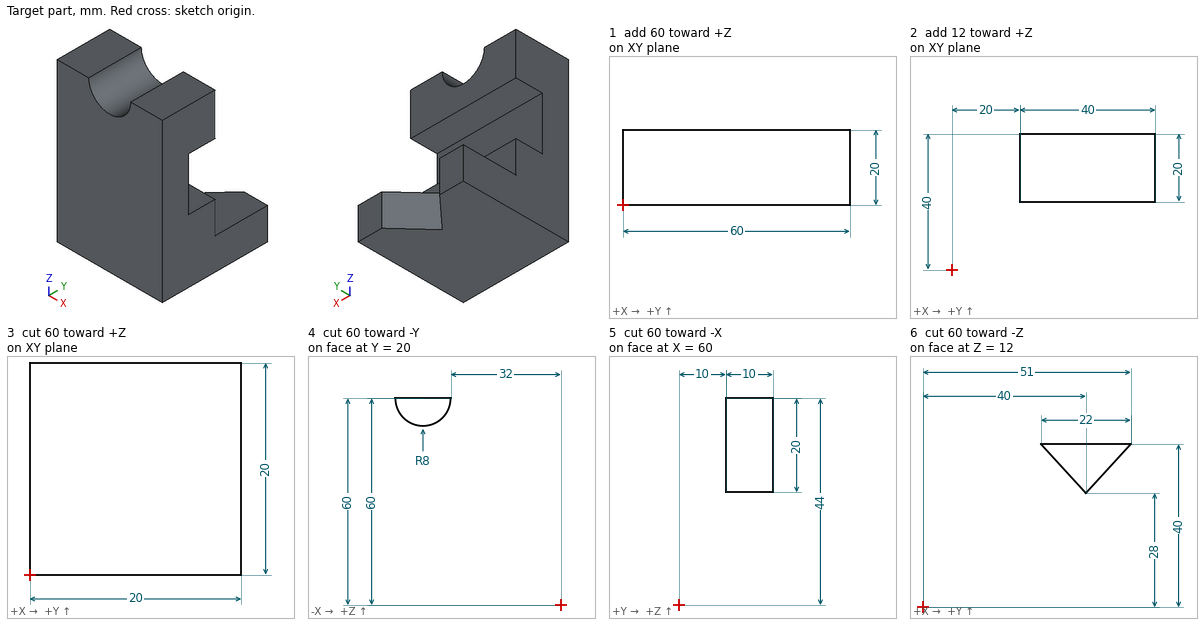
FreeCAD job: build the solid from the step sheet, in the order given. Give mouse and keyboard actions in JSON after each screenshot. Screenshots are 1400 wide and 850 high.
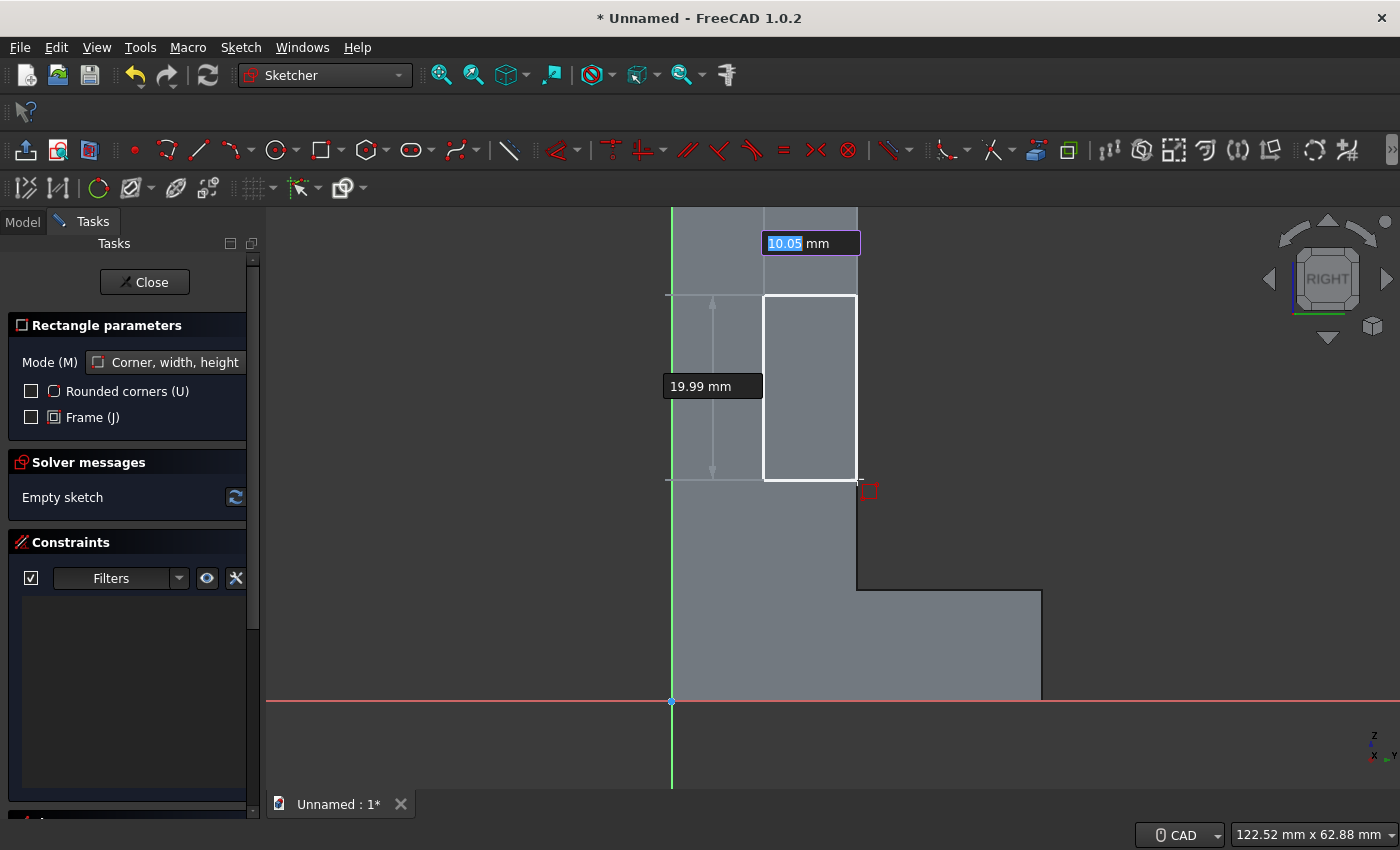
{"action": "type", "text": "10"}
{"action": "key", "text": "Tab"}
{"action": "type", "text": "20"}
{"action": "key", "text": "Return"}
{"action": "key", "text": "Escape"}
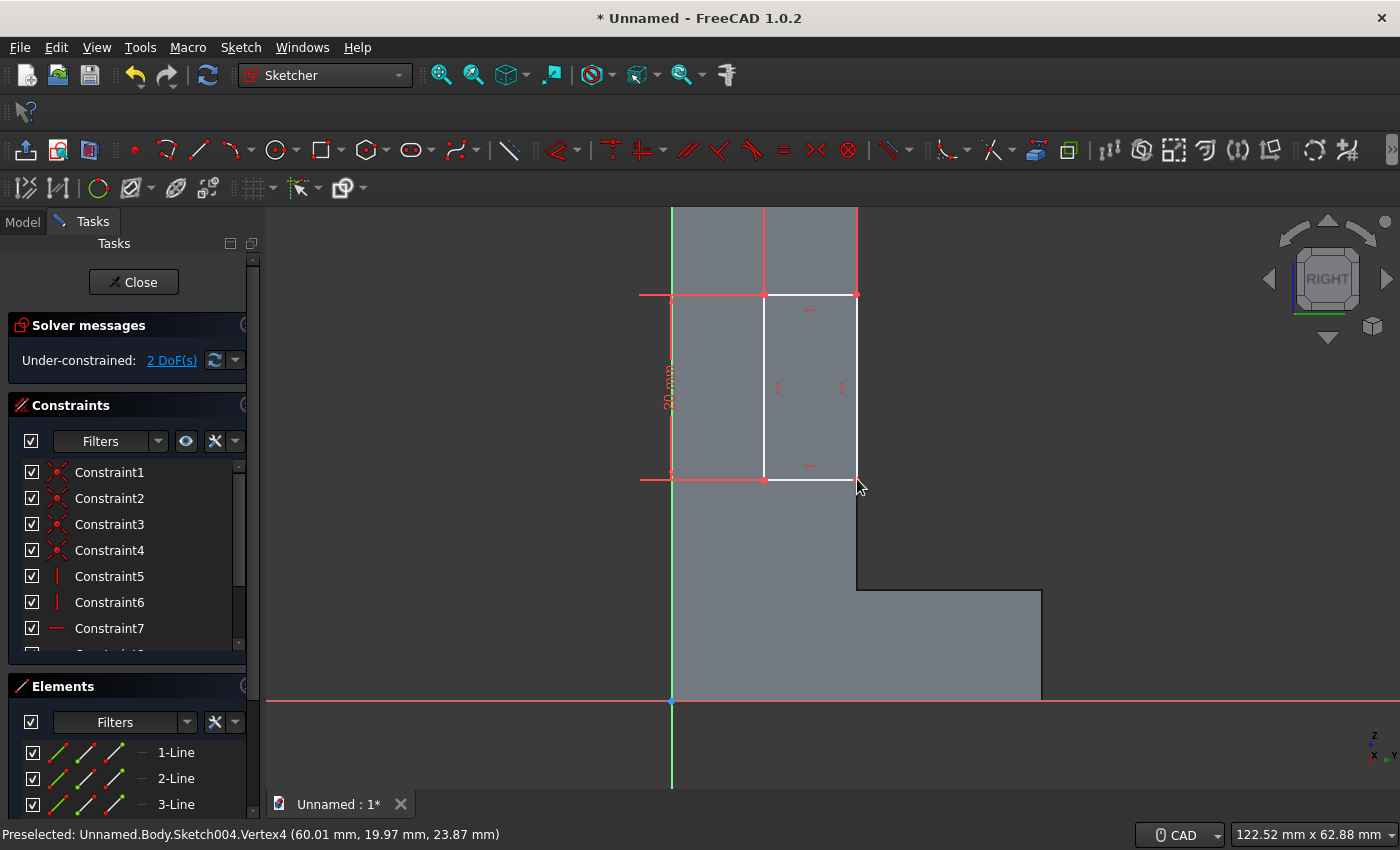
{"action": "left_click", "coordinate": [556, 150]}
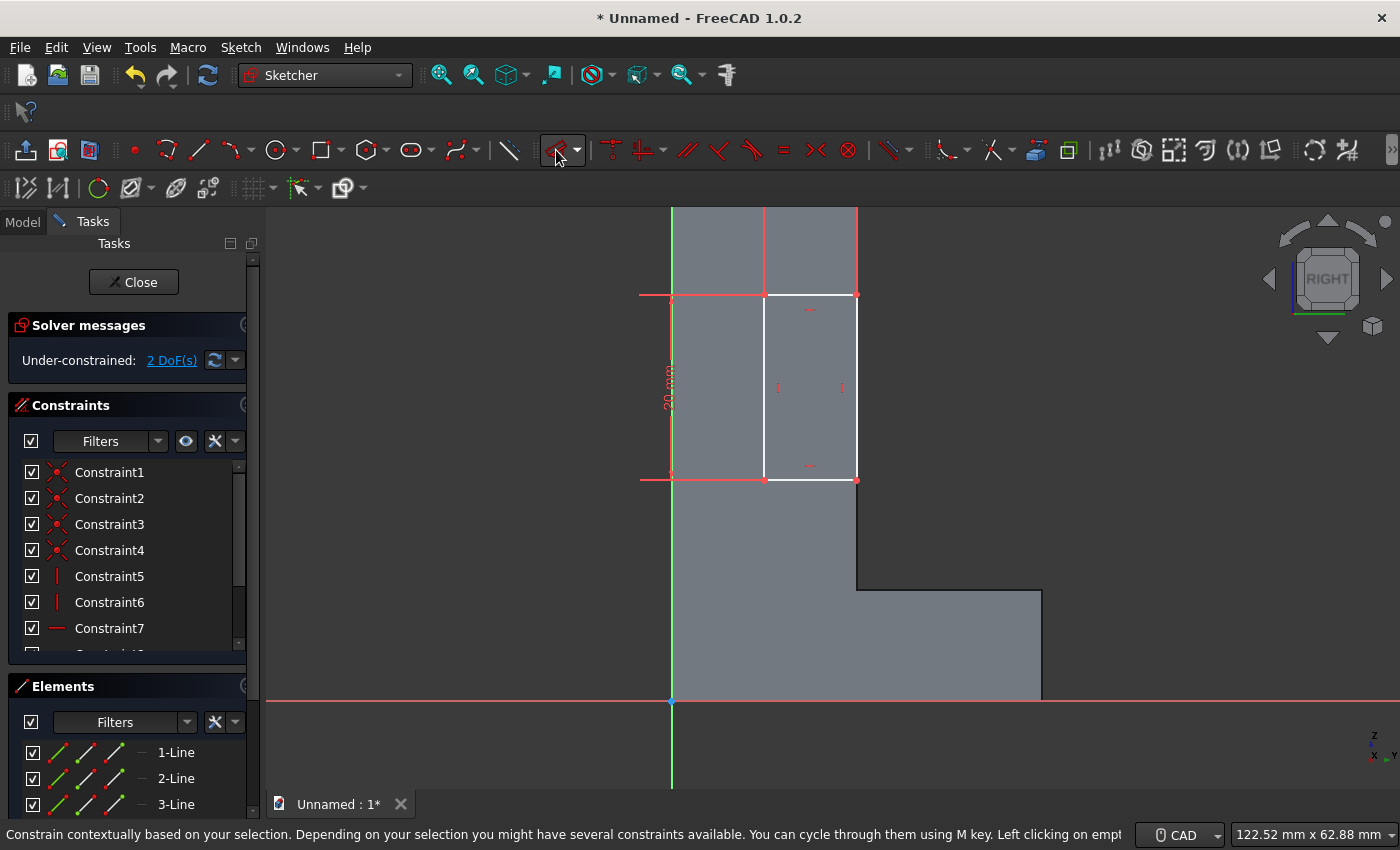
{"action": "left_click", "coordinate": [764, 295]}
{"action": "left_click", "coordinate": [718, 735]}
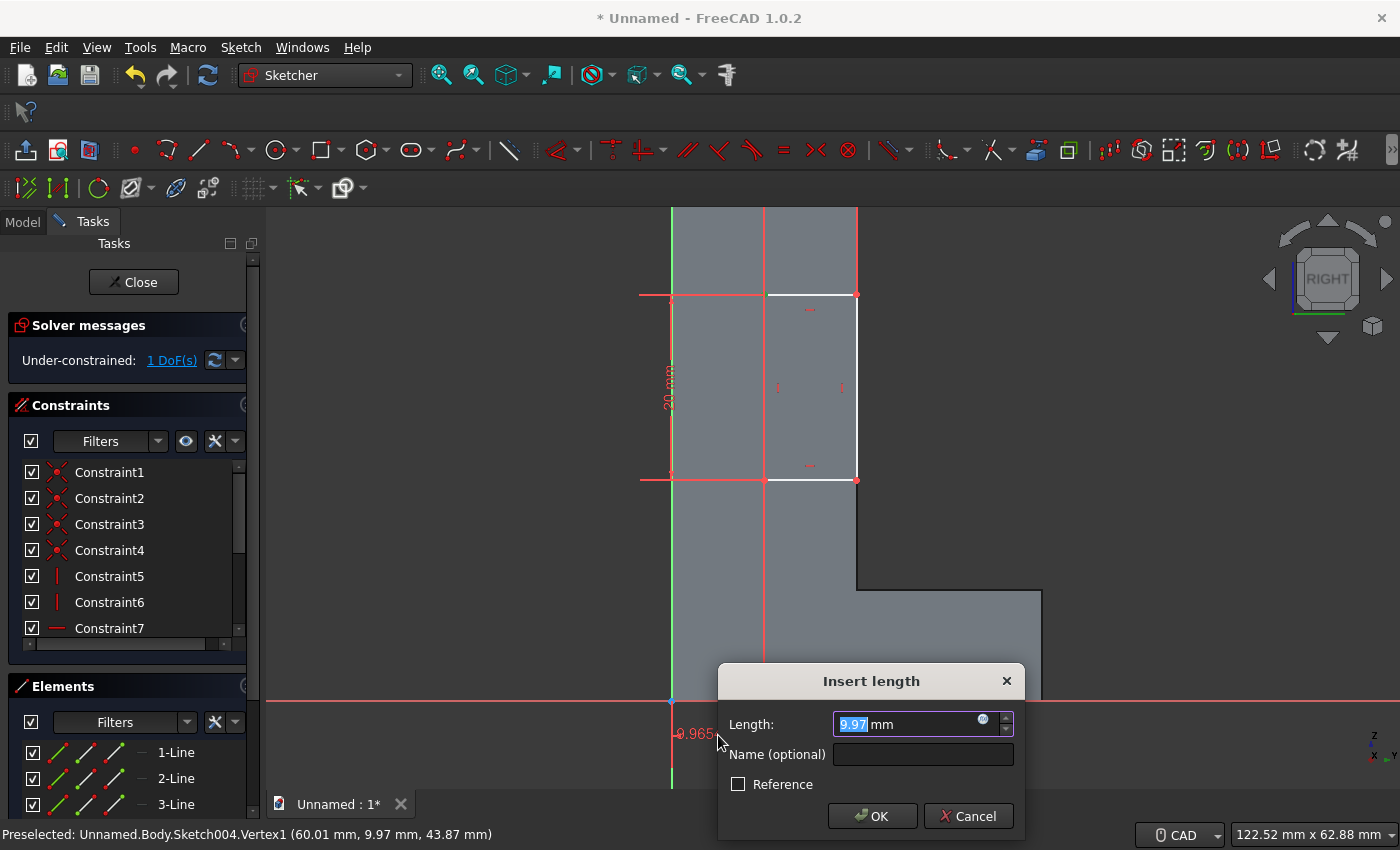
{"action": "type", "text": "10"}
{"action": "key", "text": "Return"}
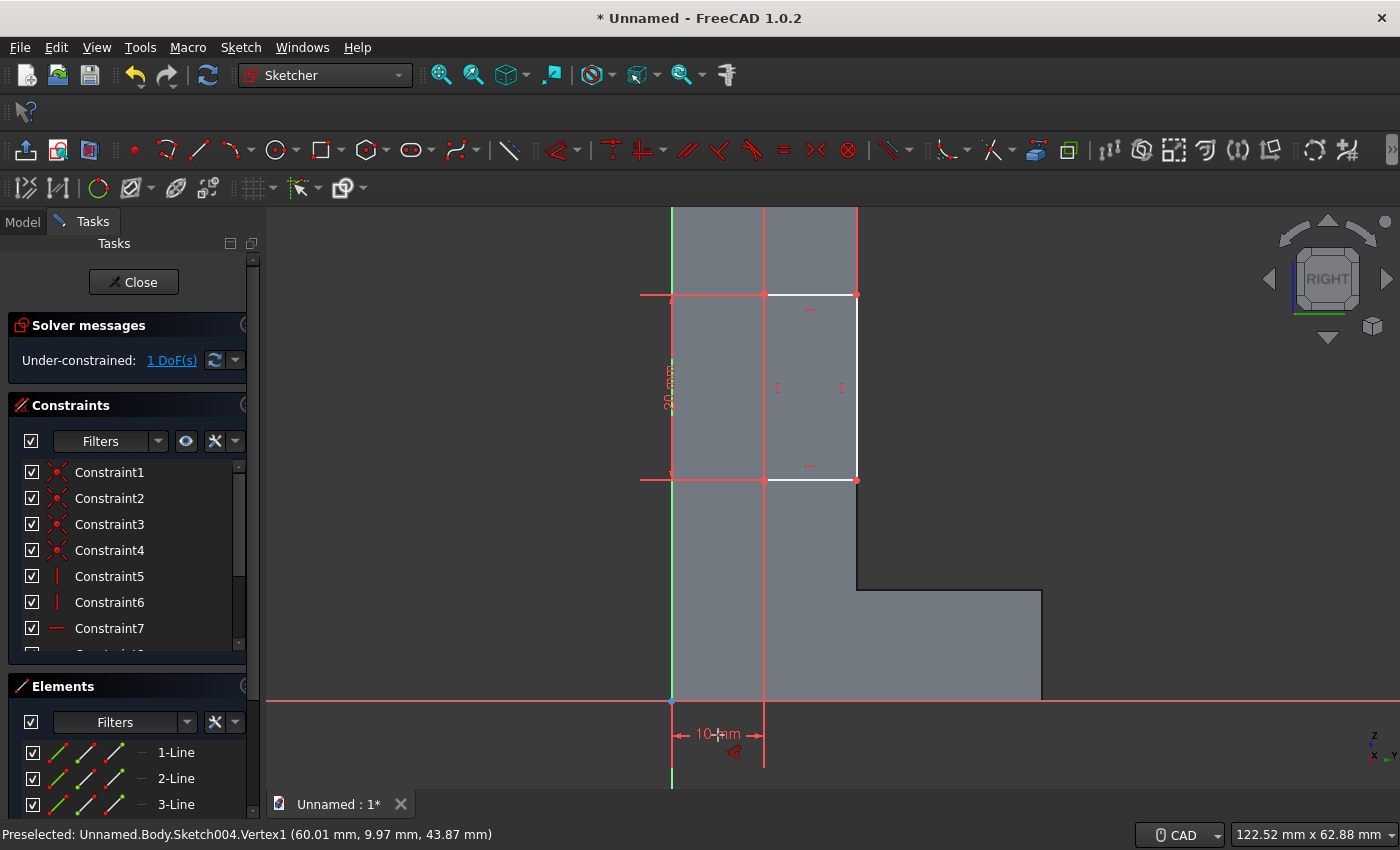
{"action": "left_click", "coordinate": [764, 295]}
{"action": "left_click", "coordinate": [638, 498]}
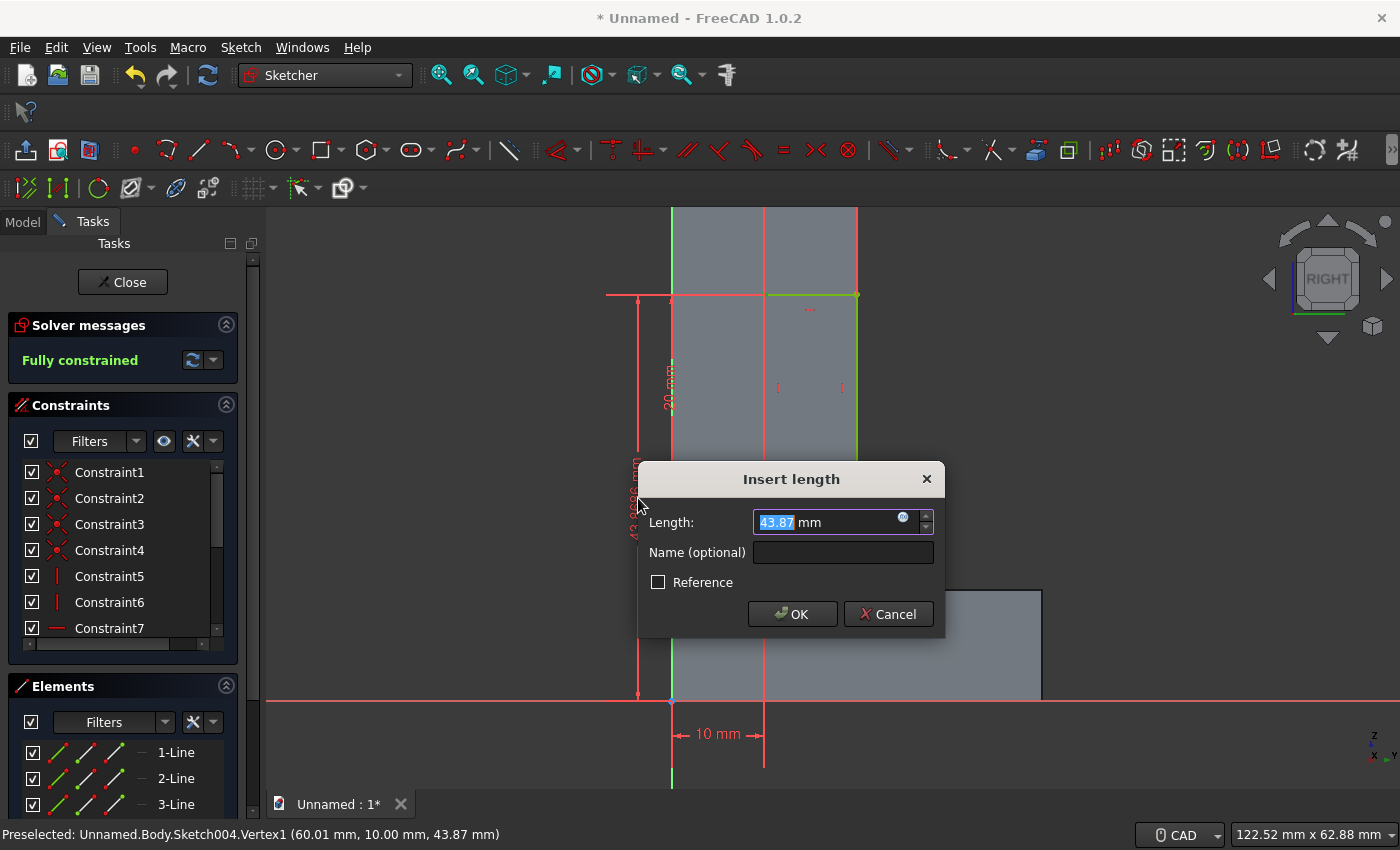
{"action": "type", "text": "44"}
{"action": "key", "text": "Return"}
{"action": "key", "text": "Escape"}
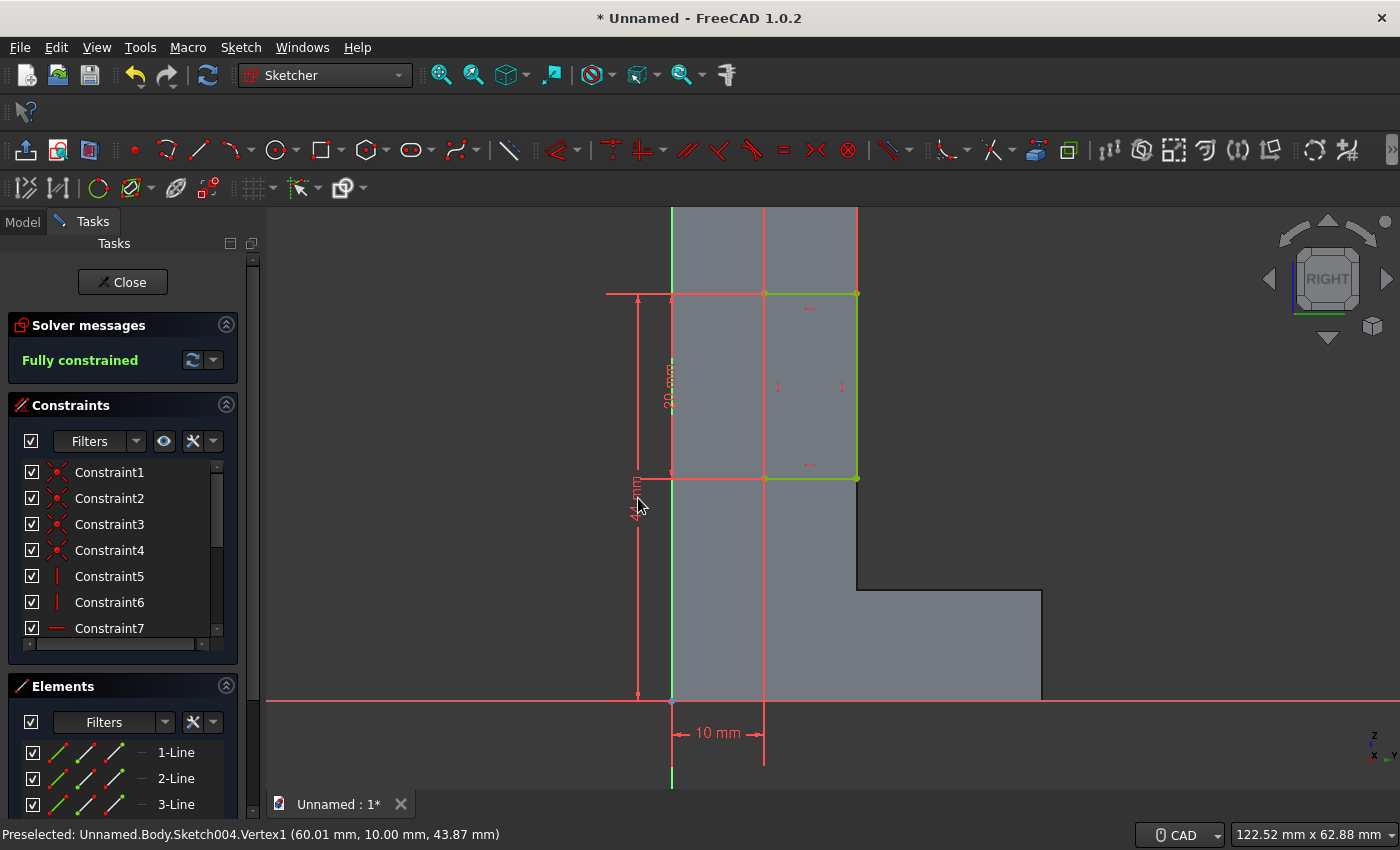
{"action": "left_click", "coordinate": [123, 282]}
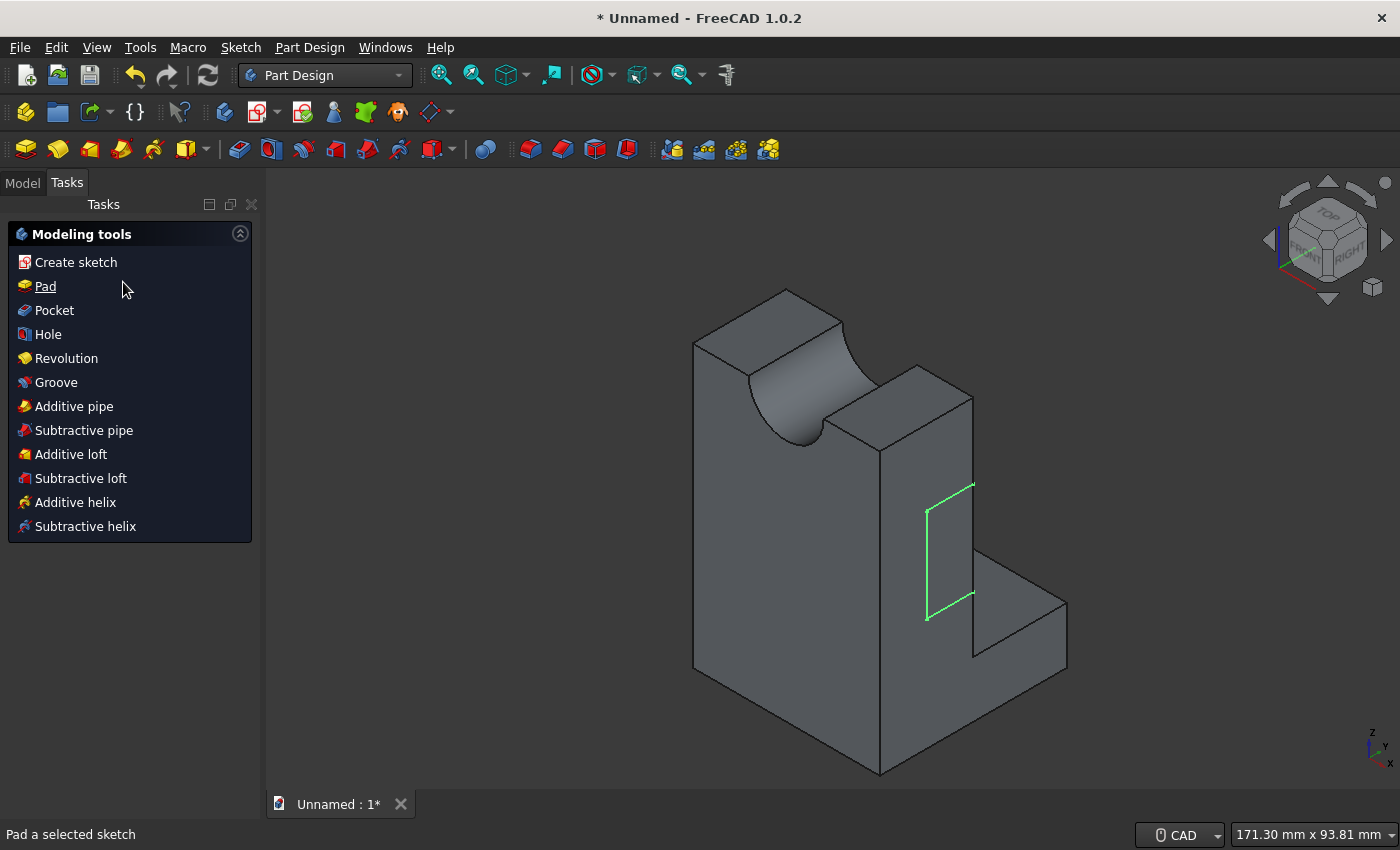
{"action": "left_click", "coordinate": [240, 150]}